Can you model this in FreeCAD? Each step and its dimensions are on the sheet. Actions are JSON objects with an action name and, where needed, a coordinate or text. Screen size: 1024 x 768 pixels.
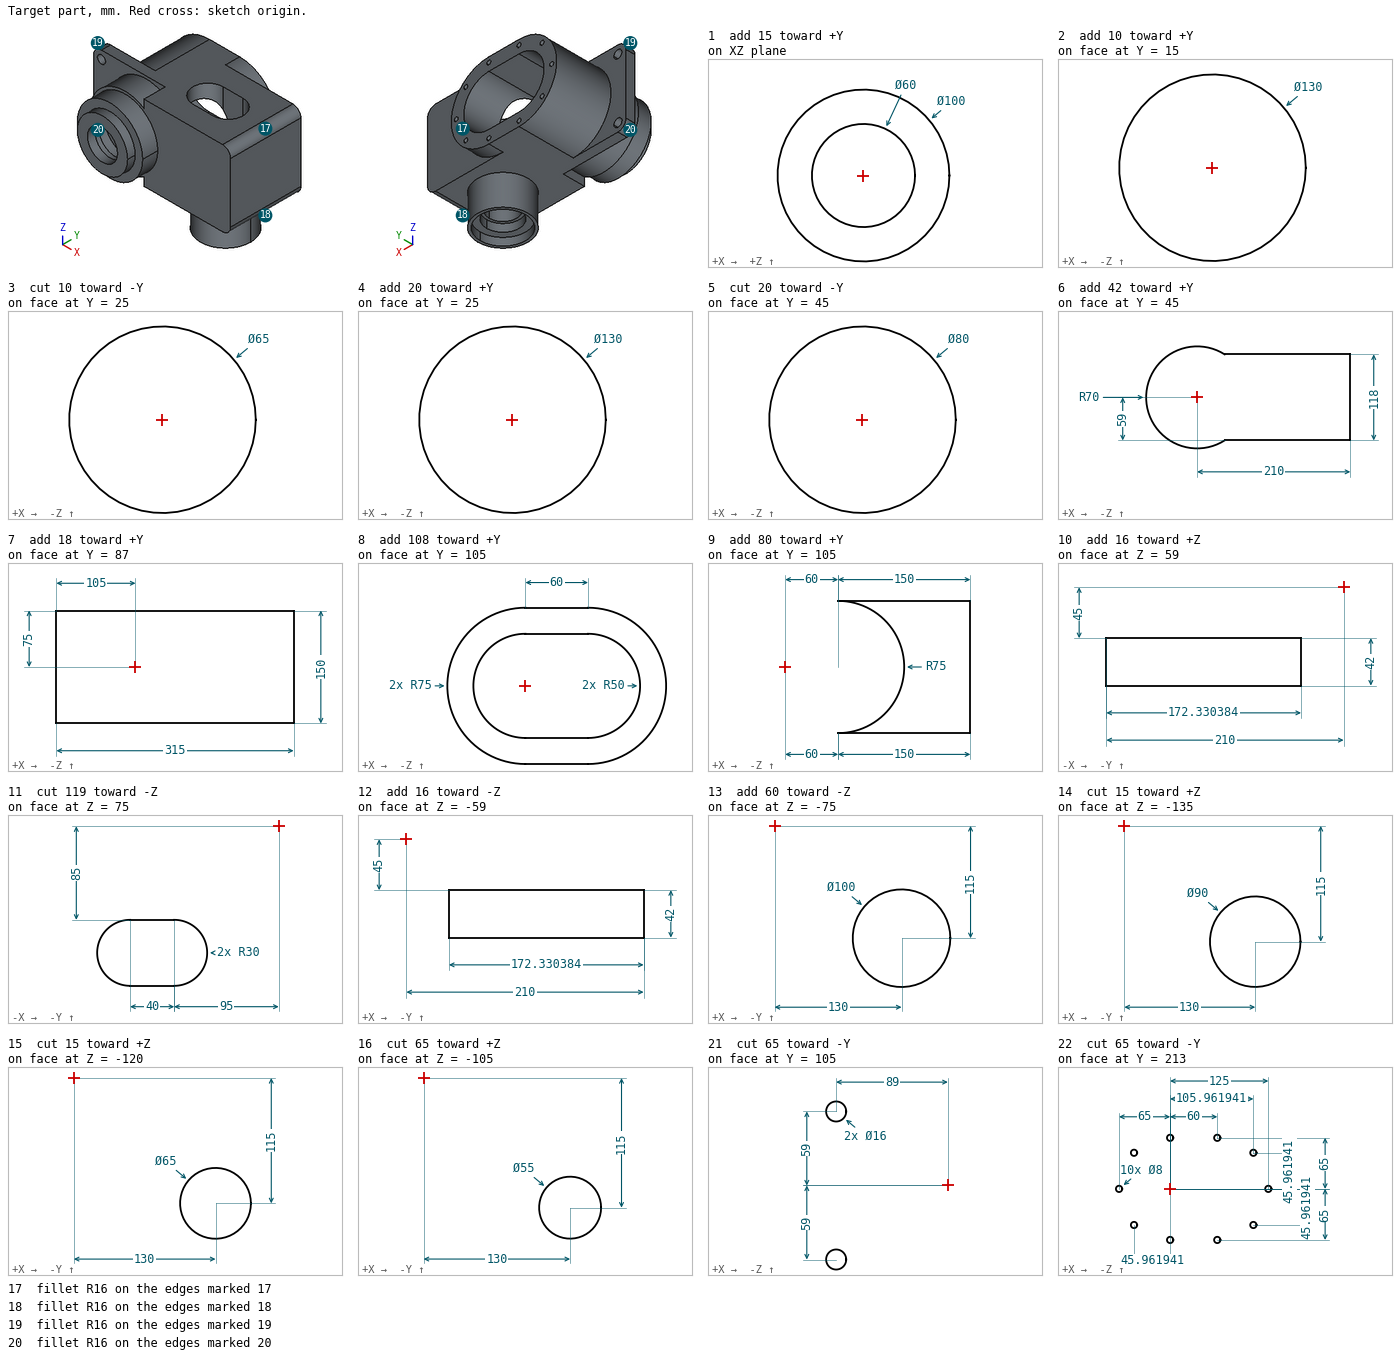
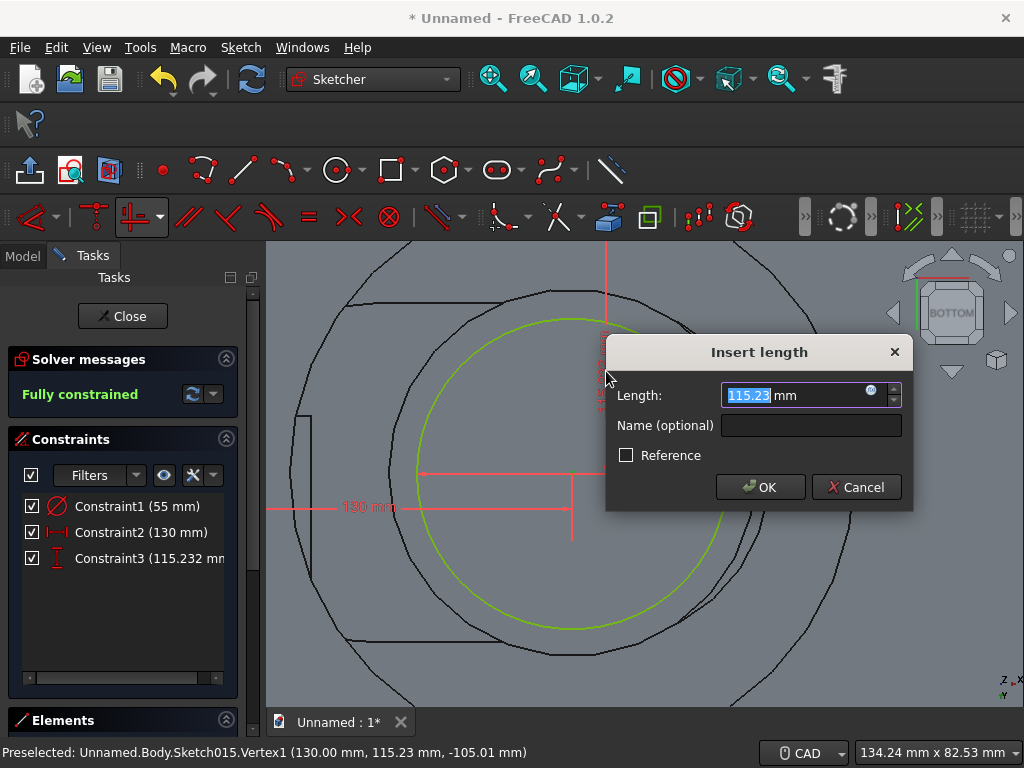
{"action": "type", "text": "115"}
{"action": "key", "text": "Return"}
{"action": "key", "text": "Escape"}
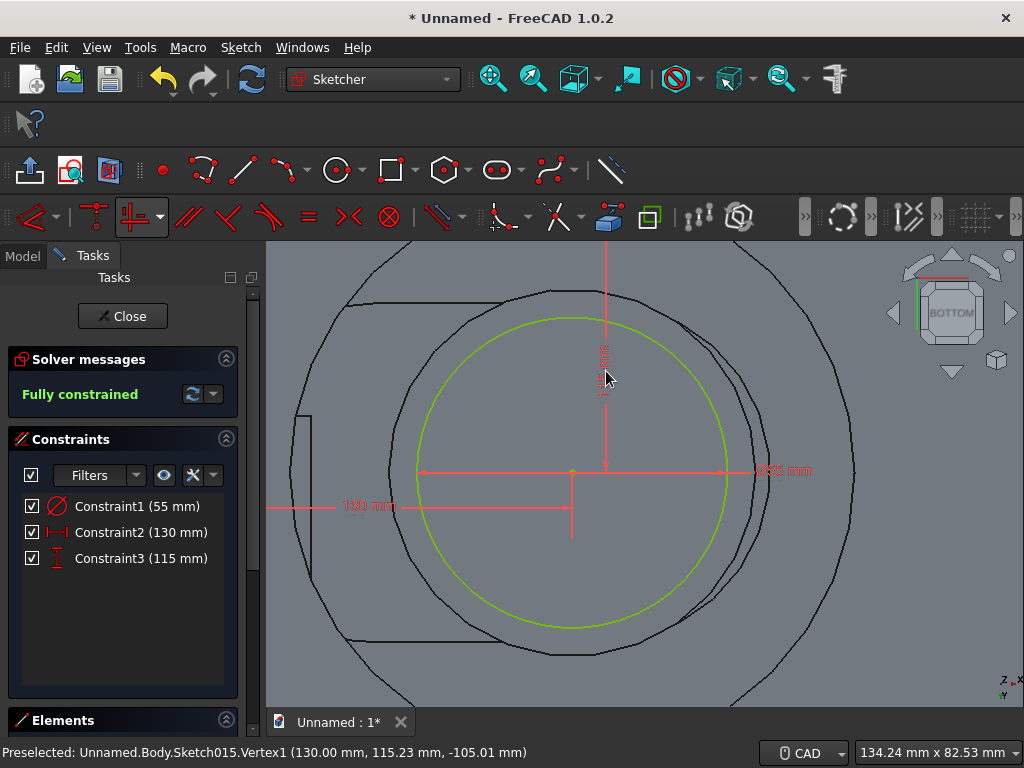
{"action": "left_click", "coordinate": [123, 316]}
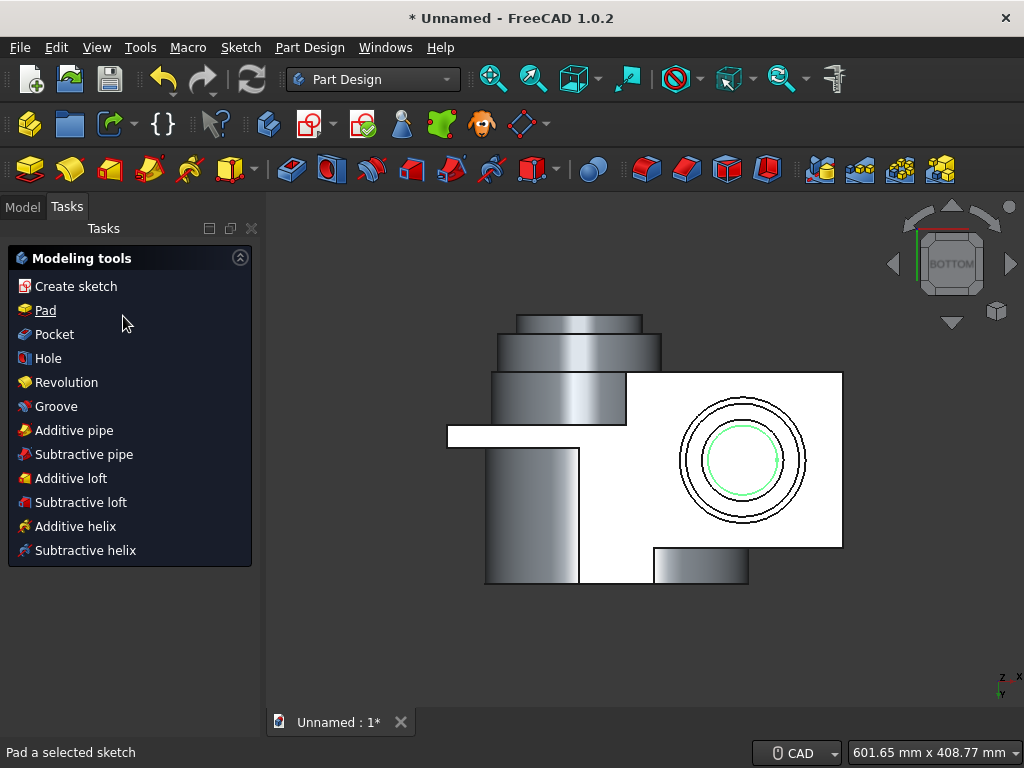
{"action": "left_click", "coordinate": [292, 170]}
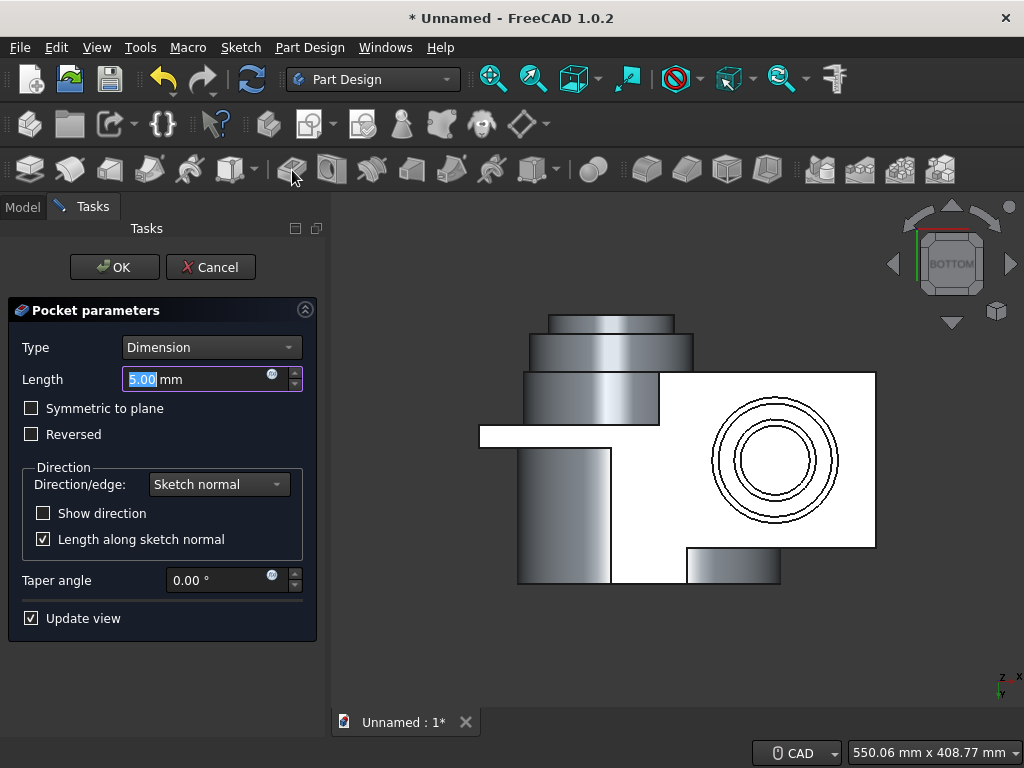
{"action": "type", "text": "65"}
{"action": "key", "text": "Tab"}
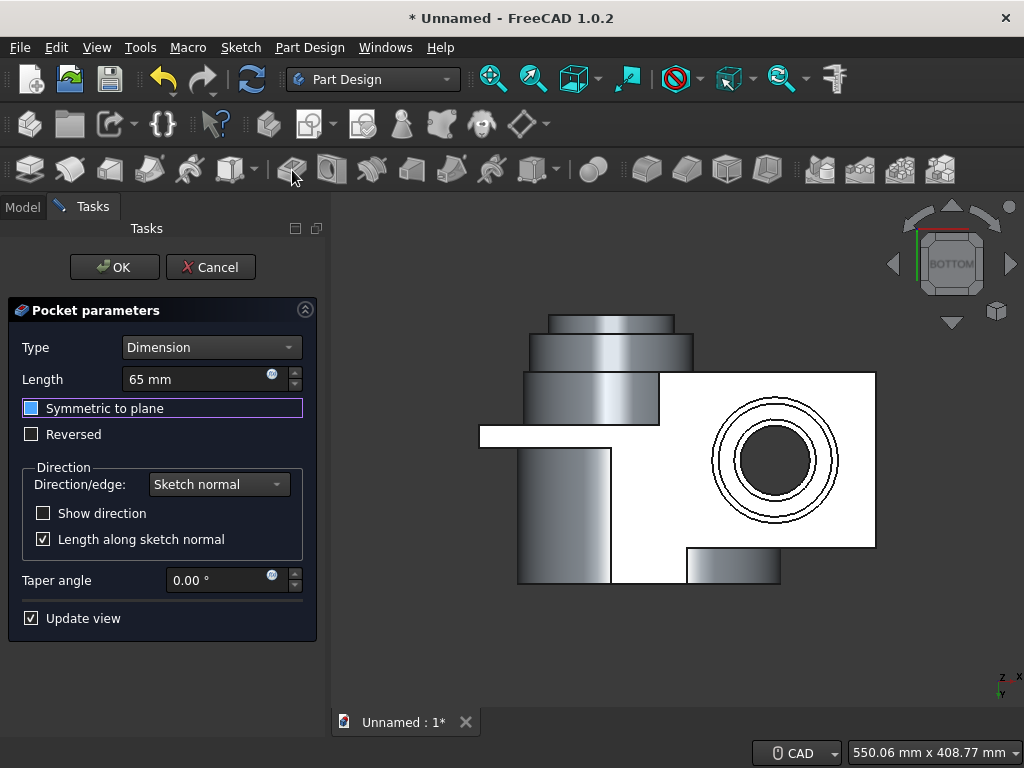
{"action": "left_click", "coordinate": [115, 267]}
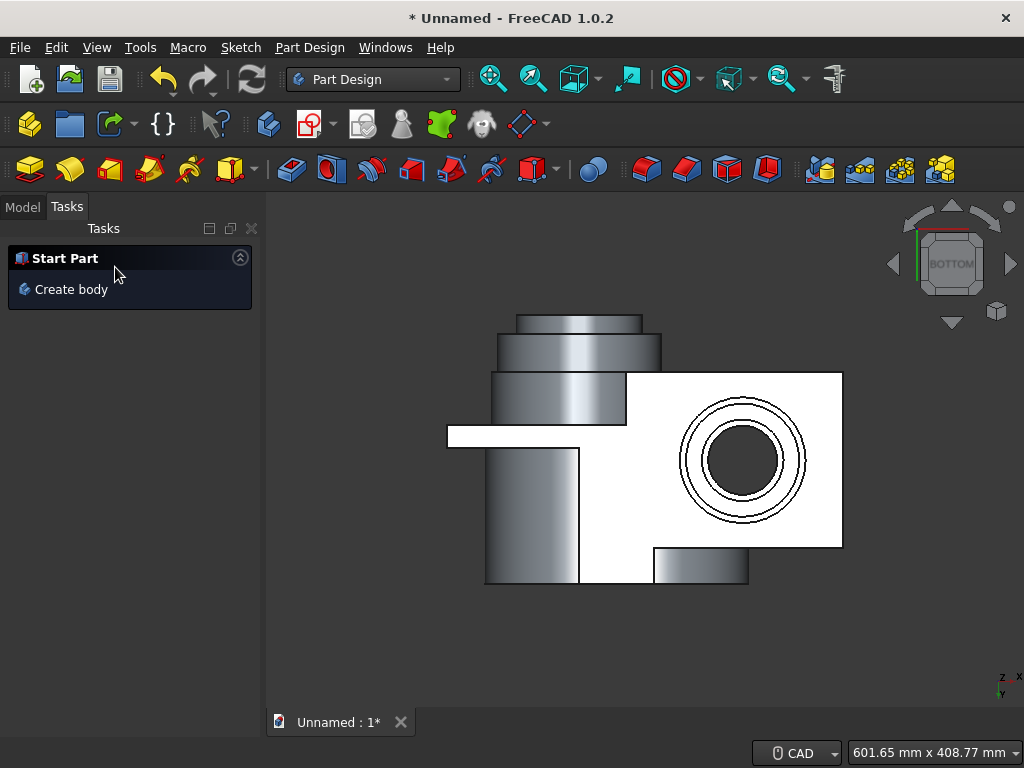
{"action": "key", "text": "0"}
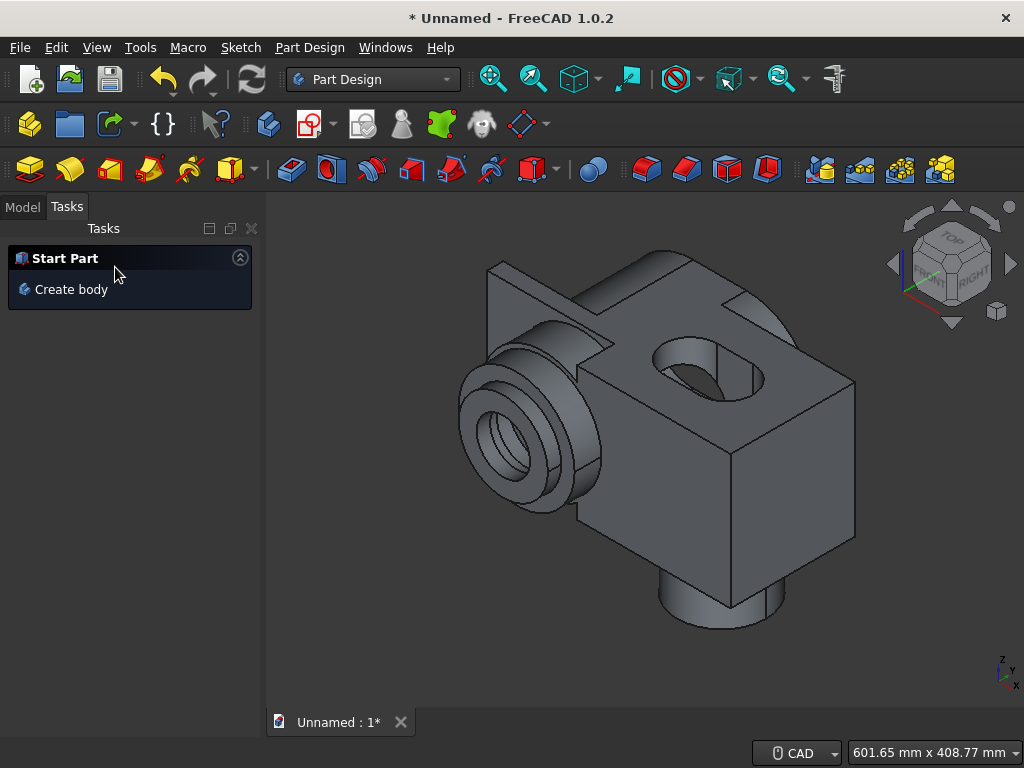
{"action": "left_click", "coordinate": [793, 417]}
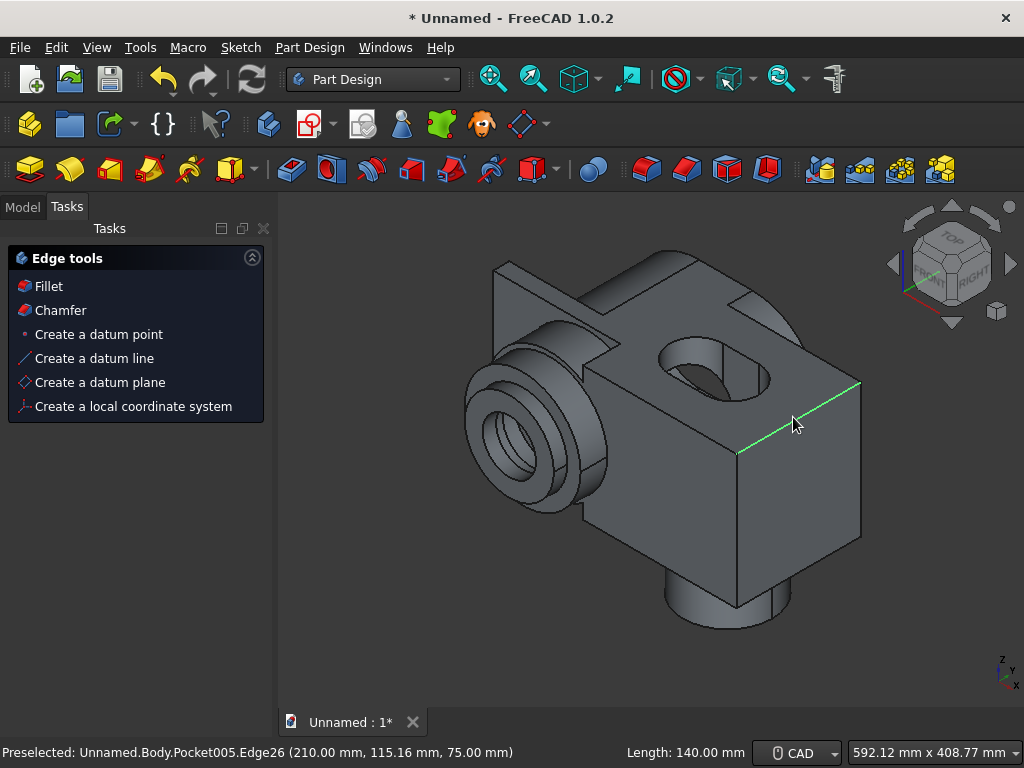
{"action": "left_click", "coordinate": [648, 170]}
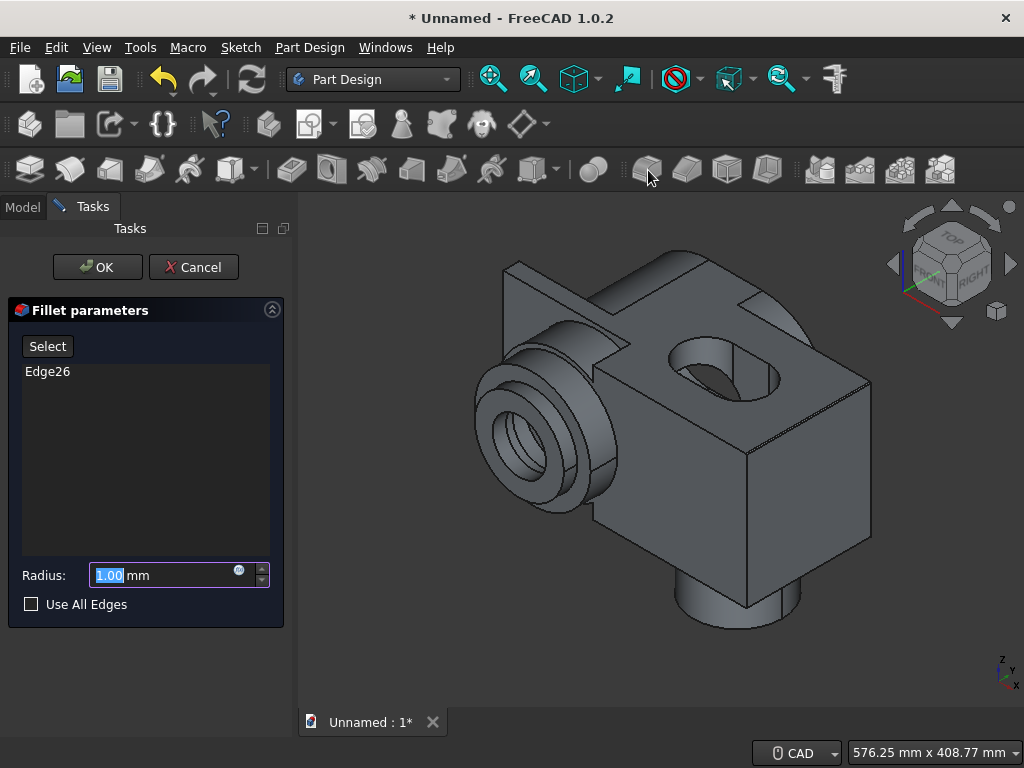
{"action": "type", "text": "16"}
{"action": "key", "text": "Tab"}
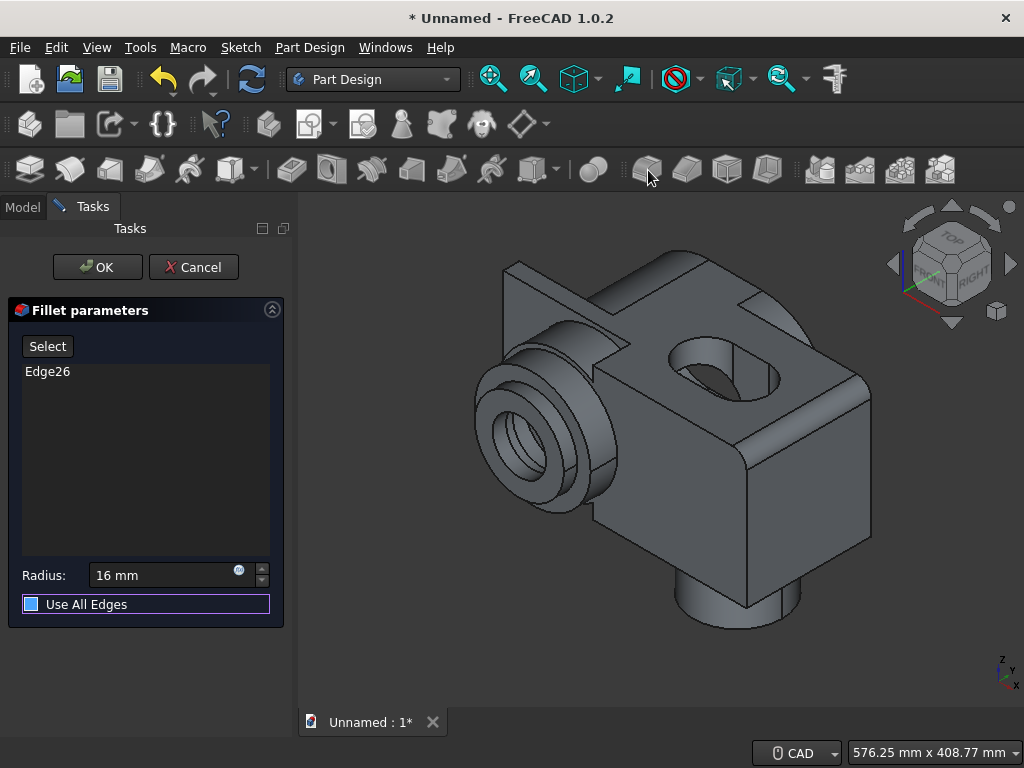
{"action": "left_click", "coordinate": [98, 267]}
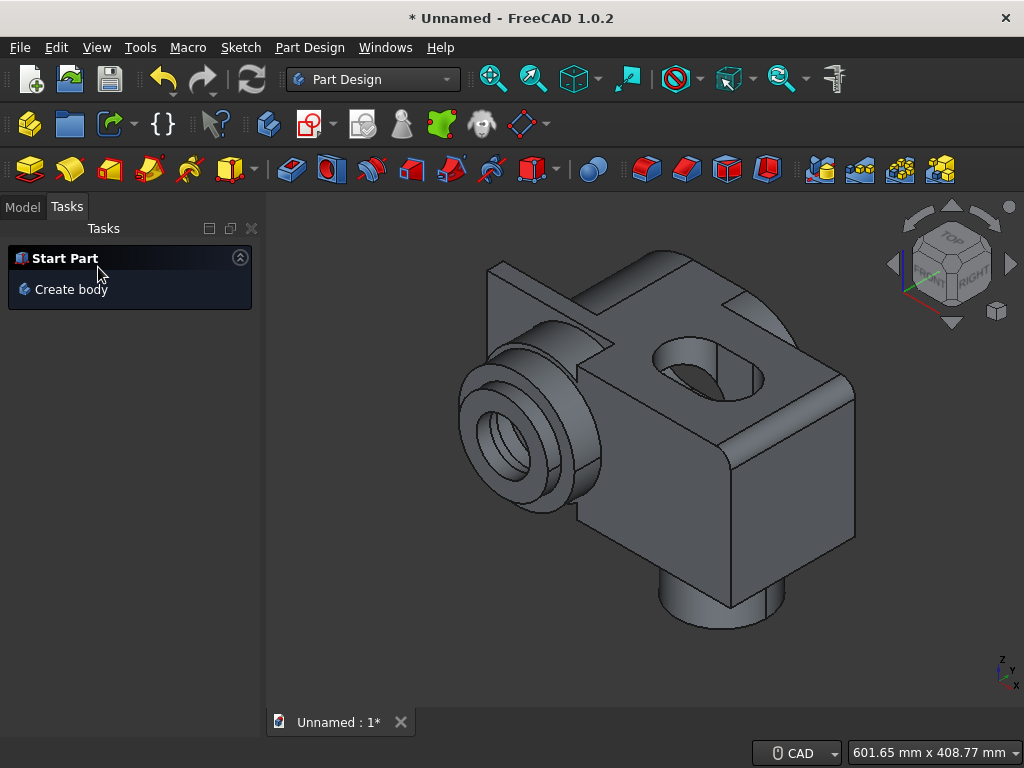
{"action": "key", "text": "2"}